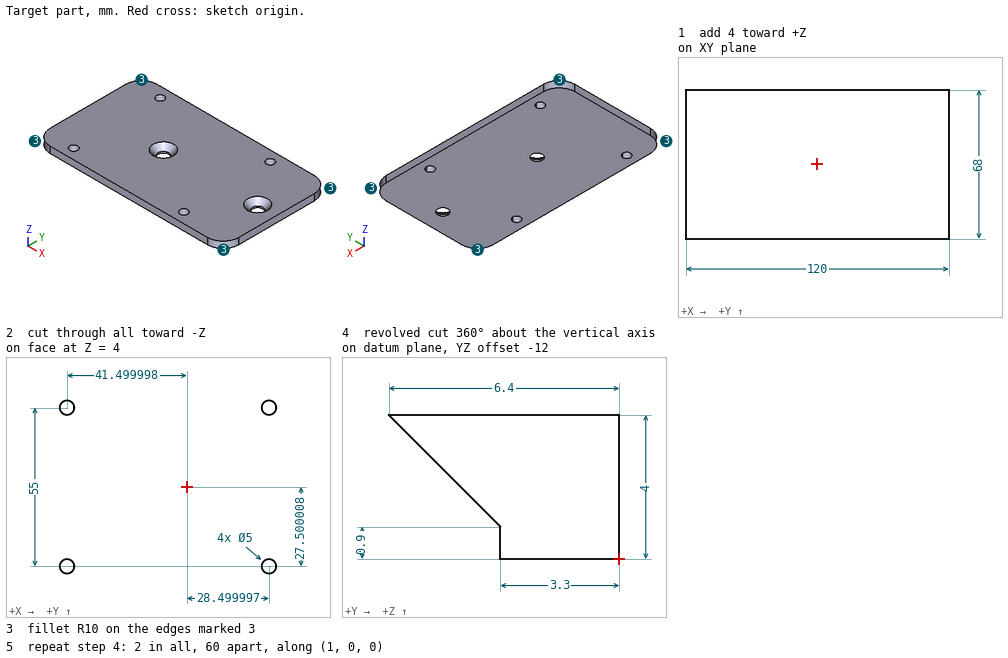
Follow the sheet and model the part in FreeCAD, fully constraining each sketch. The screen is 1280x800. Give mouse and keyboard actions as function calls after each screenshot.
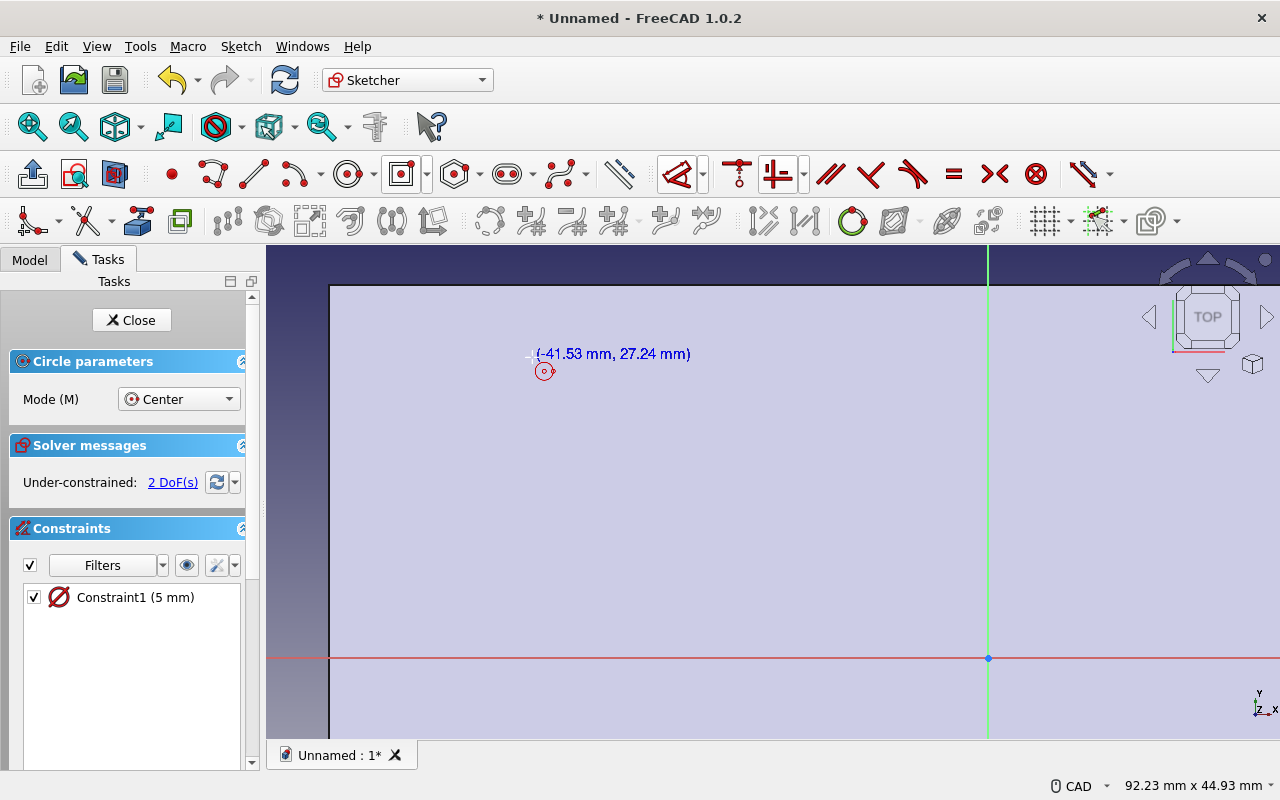
click(532, 356)
move(551, 337)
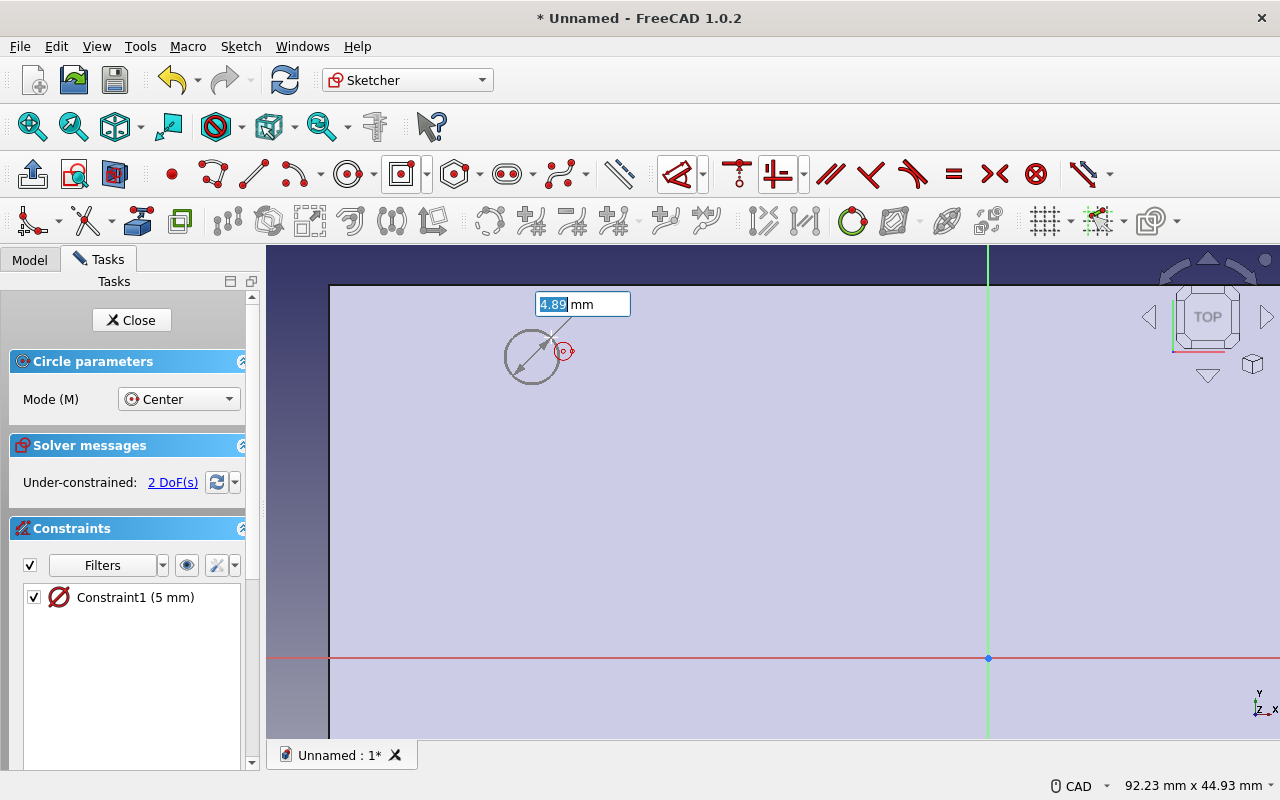
text(5)
key(Return)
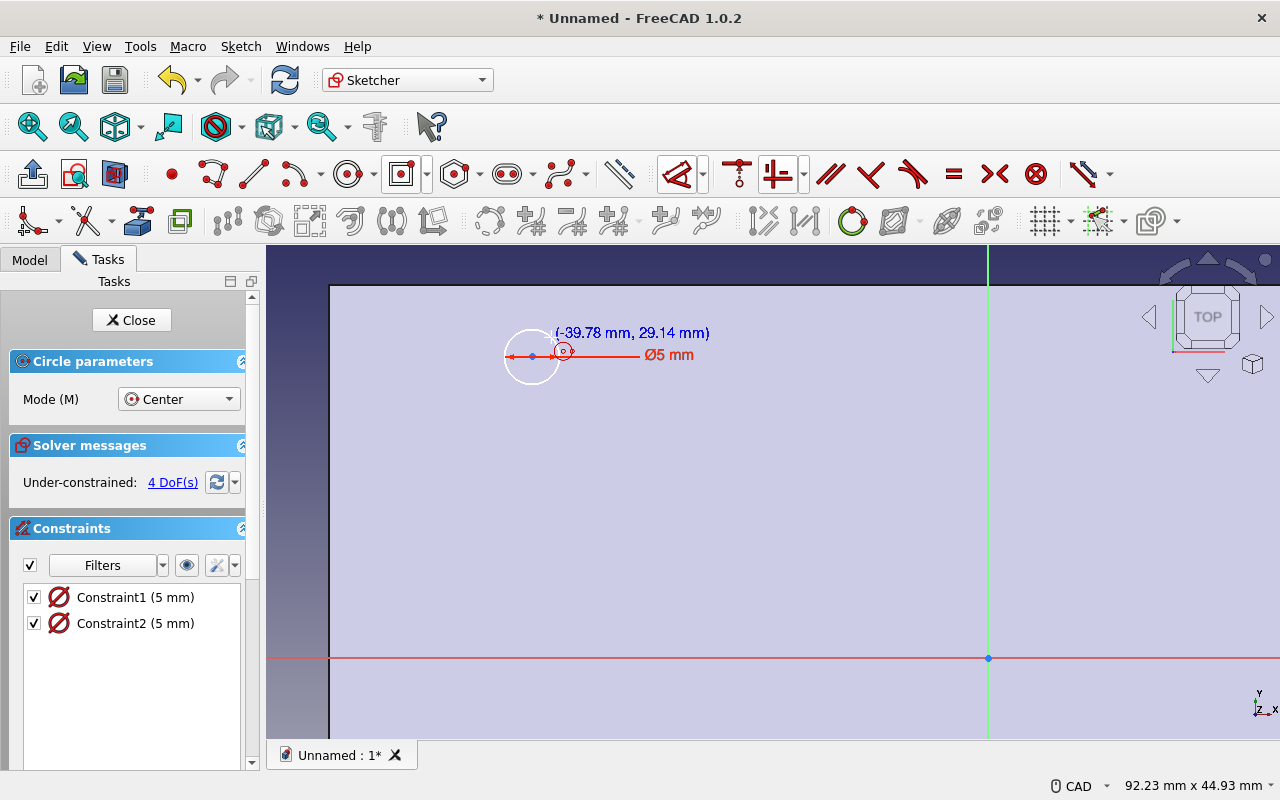
scroll(531, 356, down, 4)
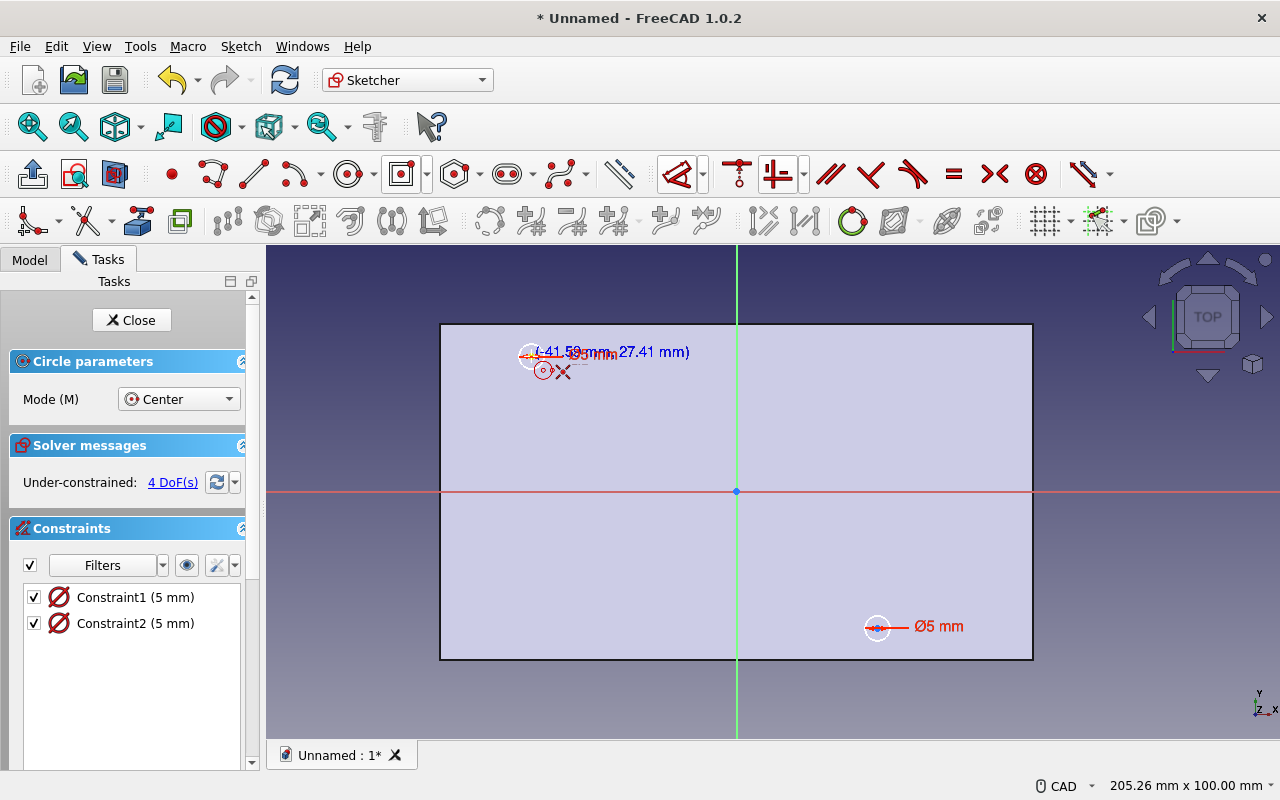
scroll(532, 628, up, 4)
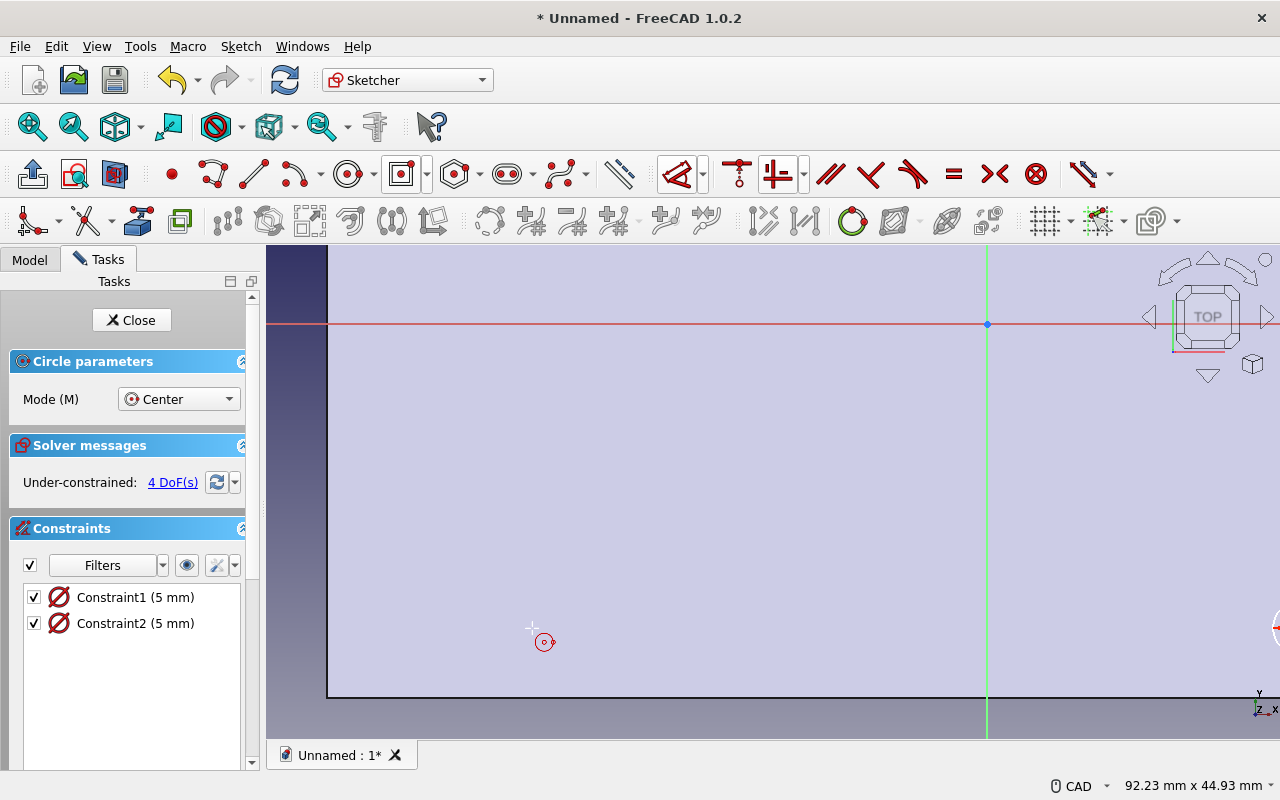
click(531, 627)
move(550, 607)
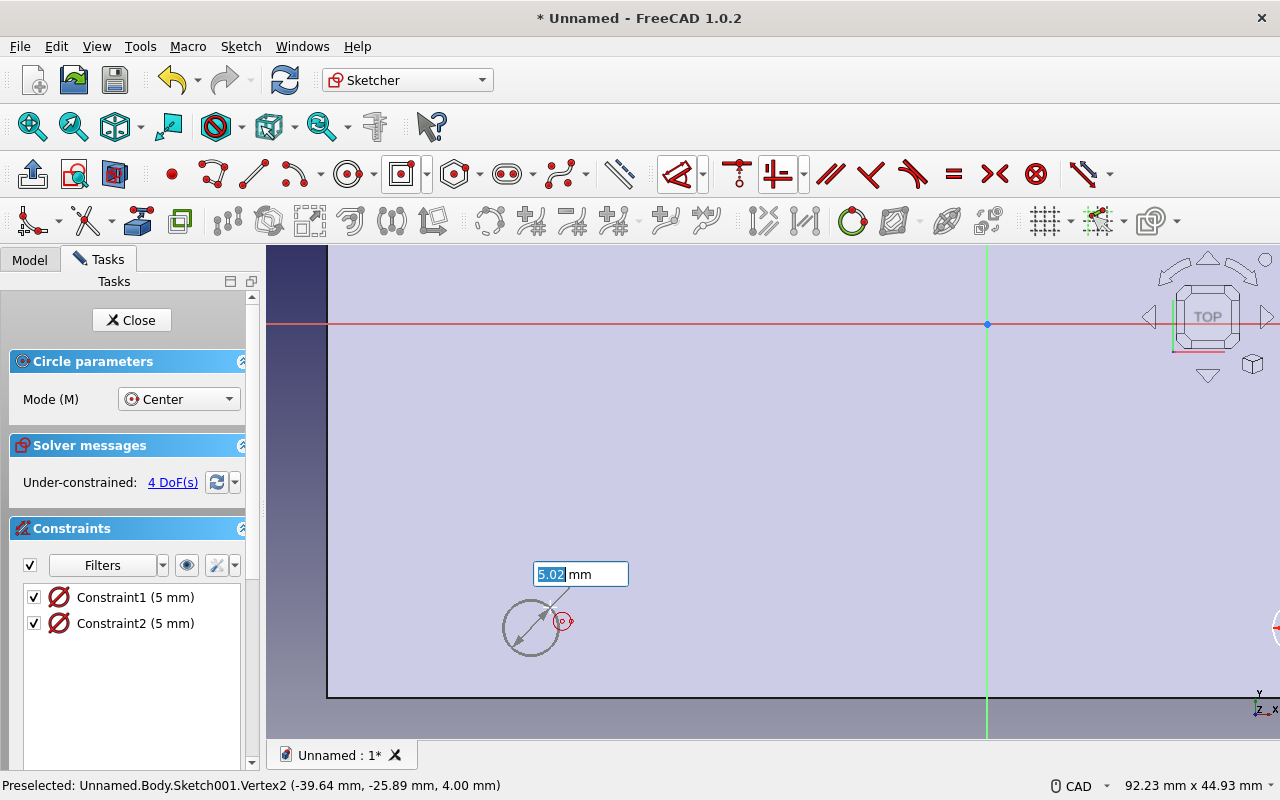
text(5)
key(Return)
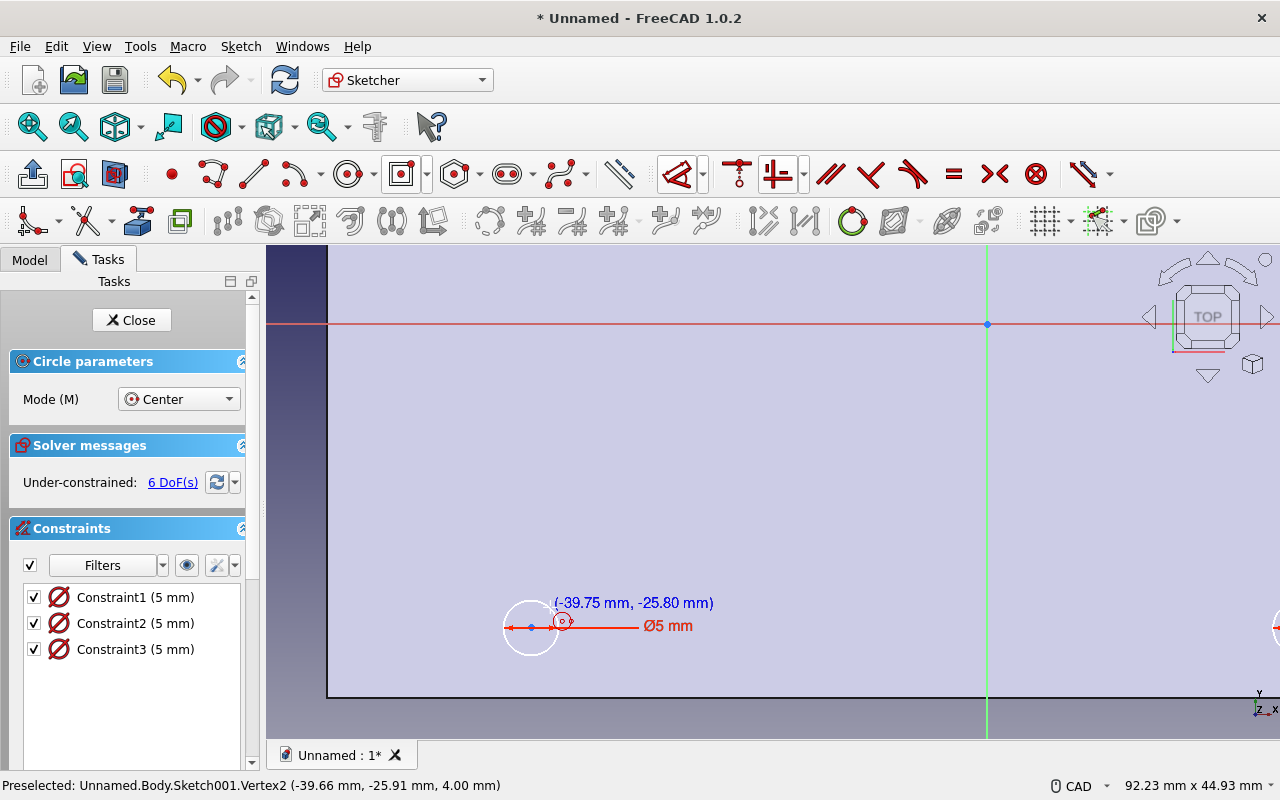
scroll(532, 629, down, 4)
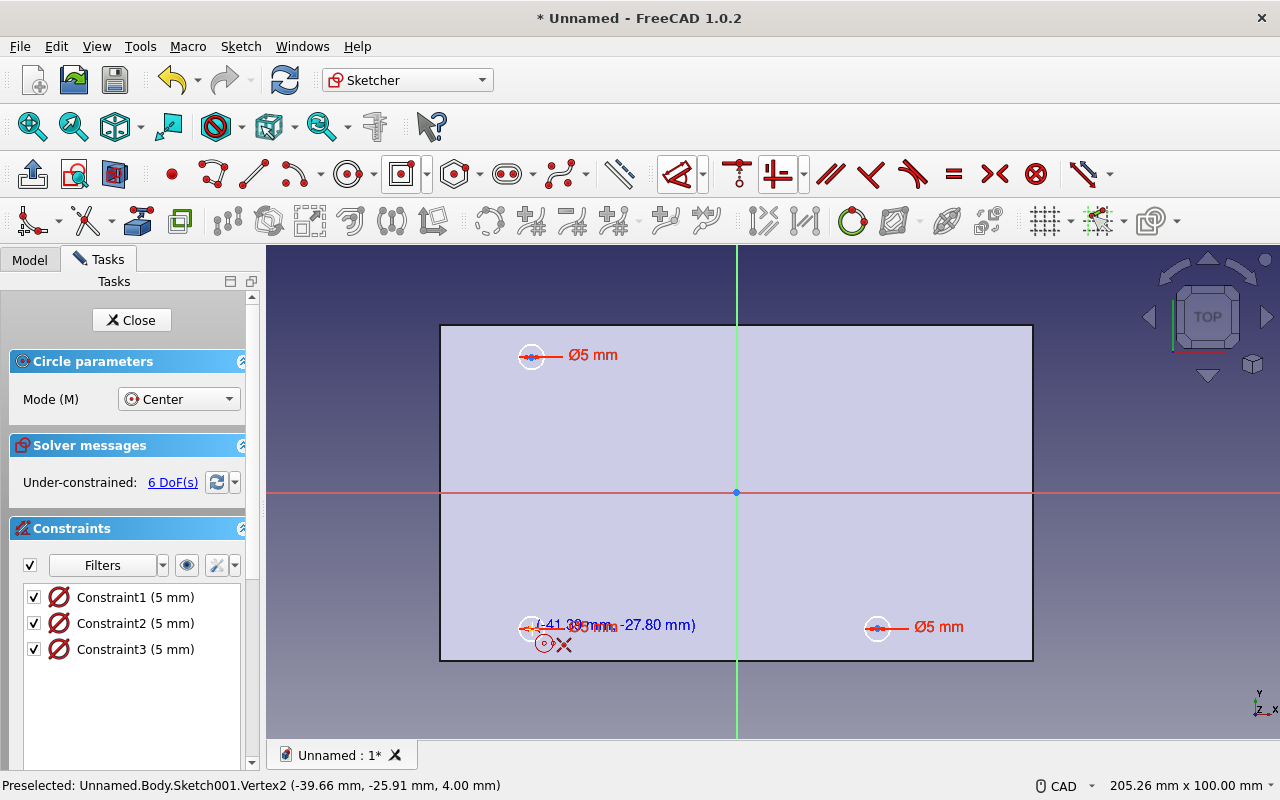
scroll(877, 357, up, 4)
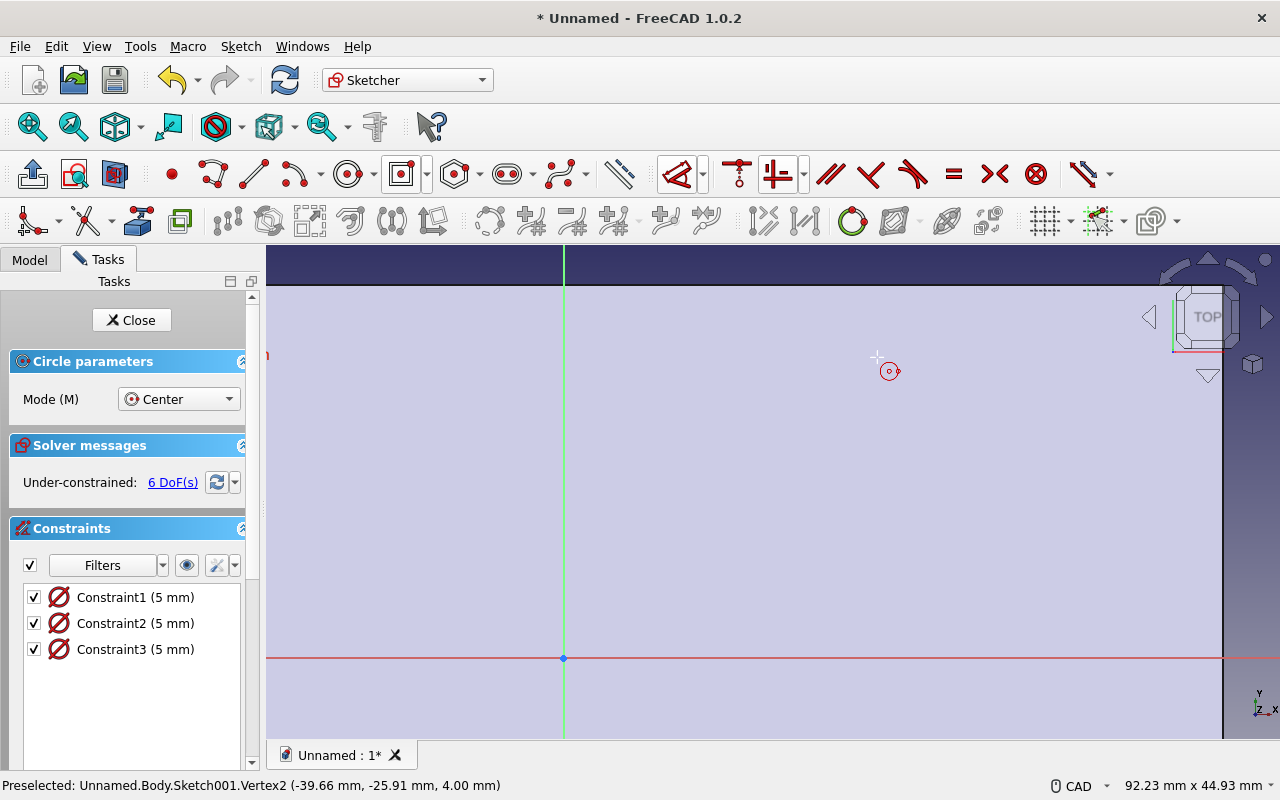
click(877, 356)
move(897, 337)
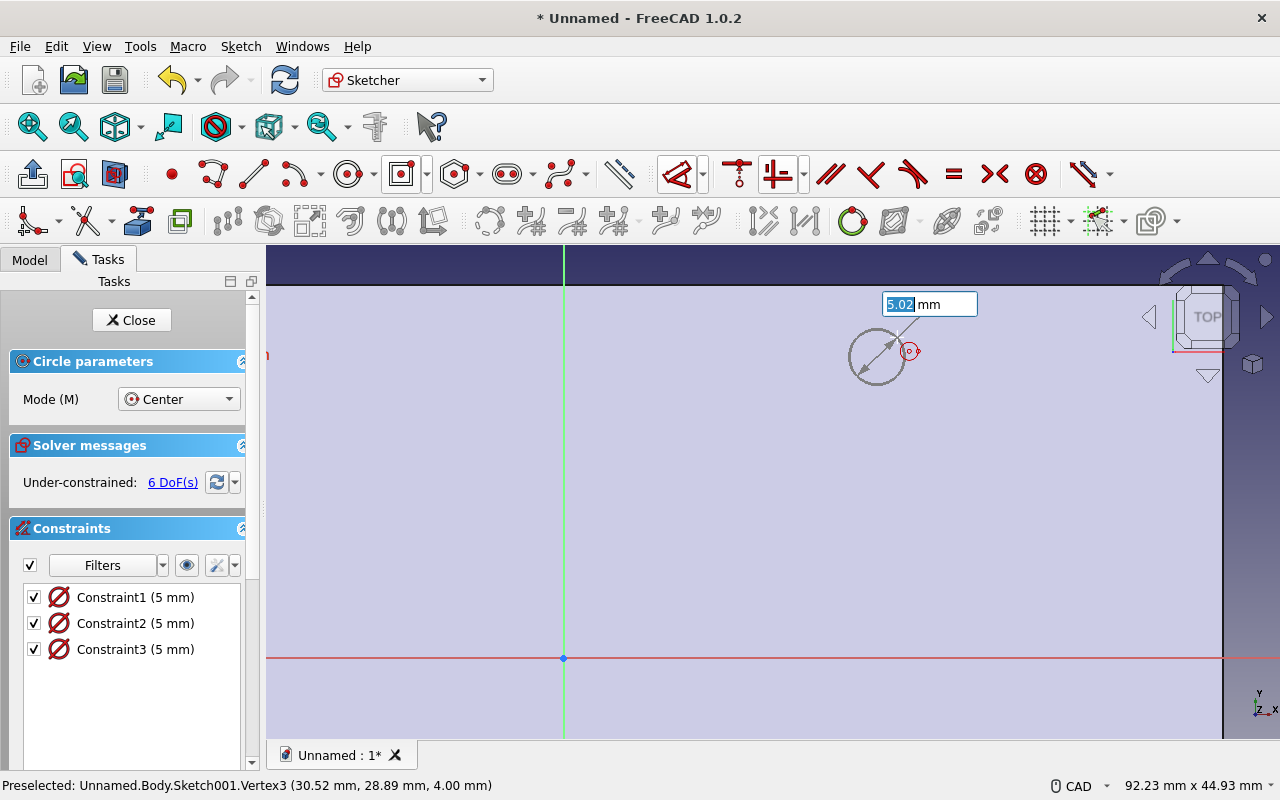
text(5)
key(Return)
key(Escape)